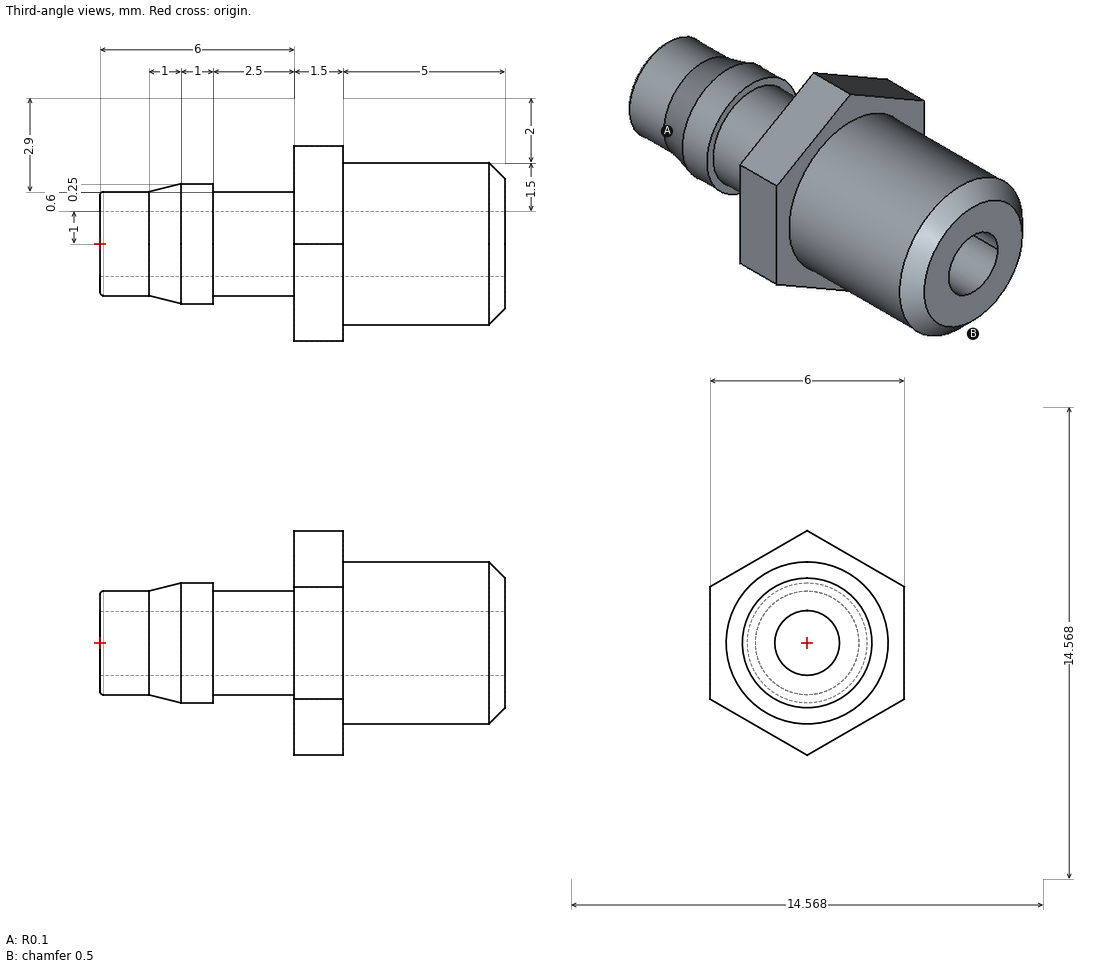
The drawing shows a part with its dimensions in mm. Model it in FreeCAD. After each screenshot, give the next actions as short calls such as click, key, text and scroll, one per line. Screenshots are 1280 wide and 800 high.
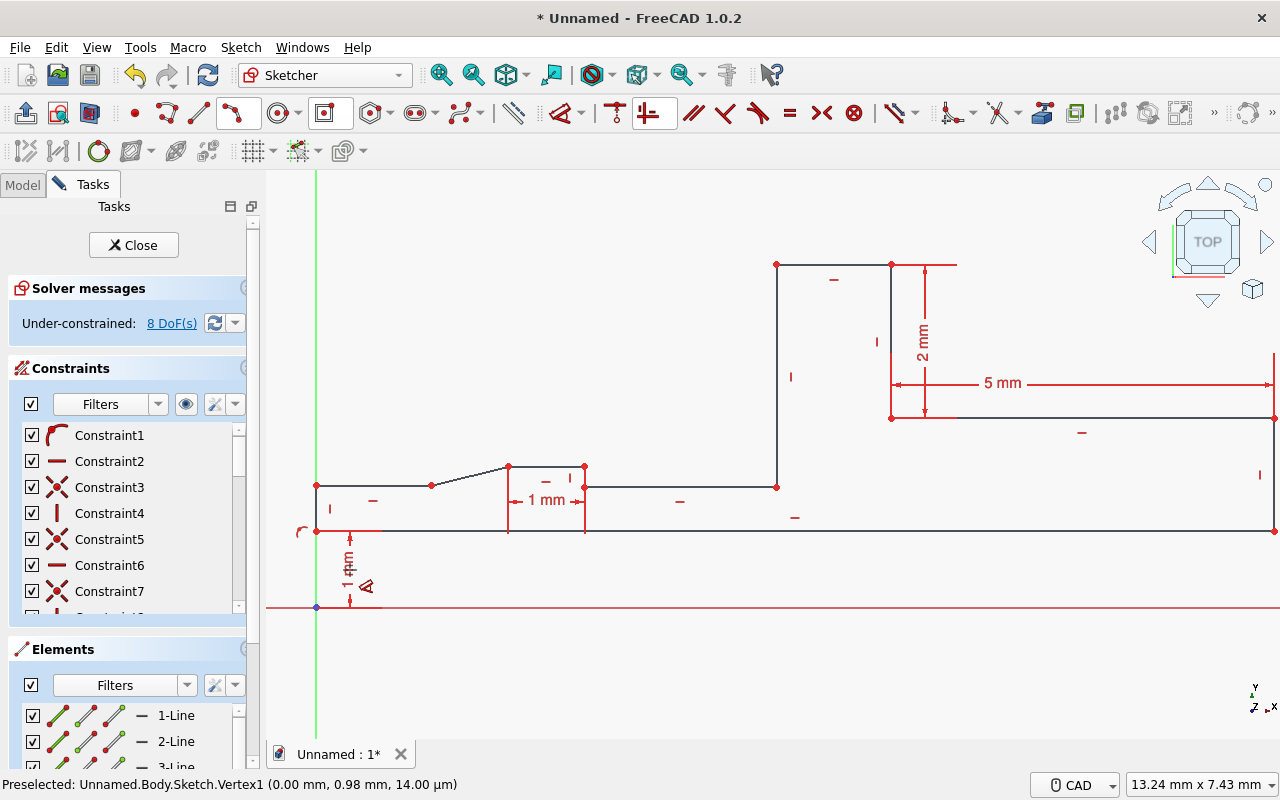
click(777, 265)
click(547, 642)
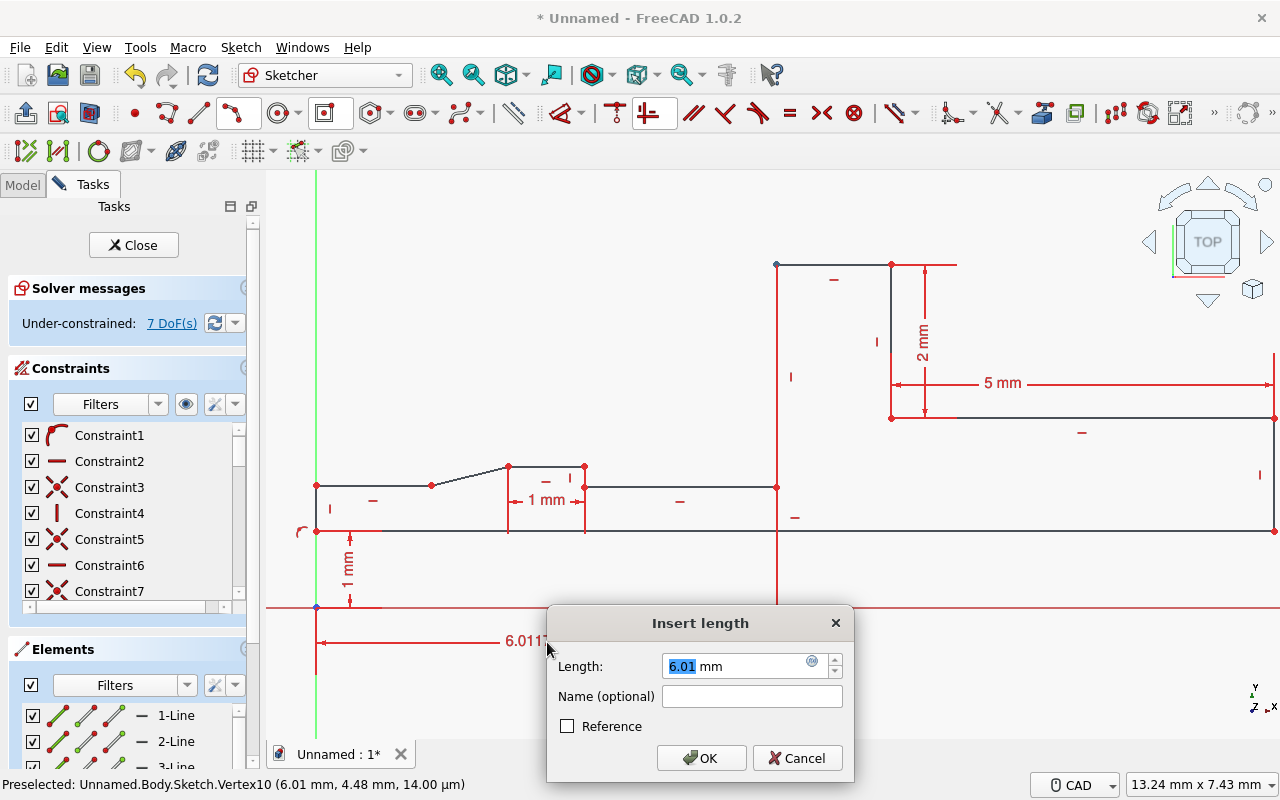
text(6)
key(Return)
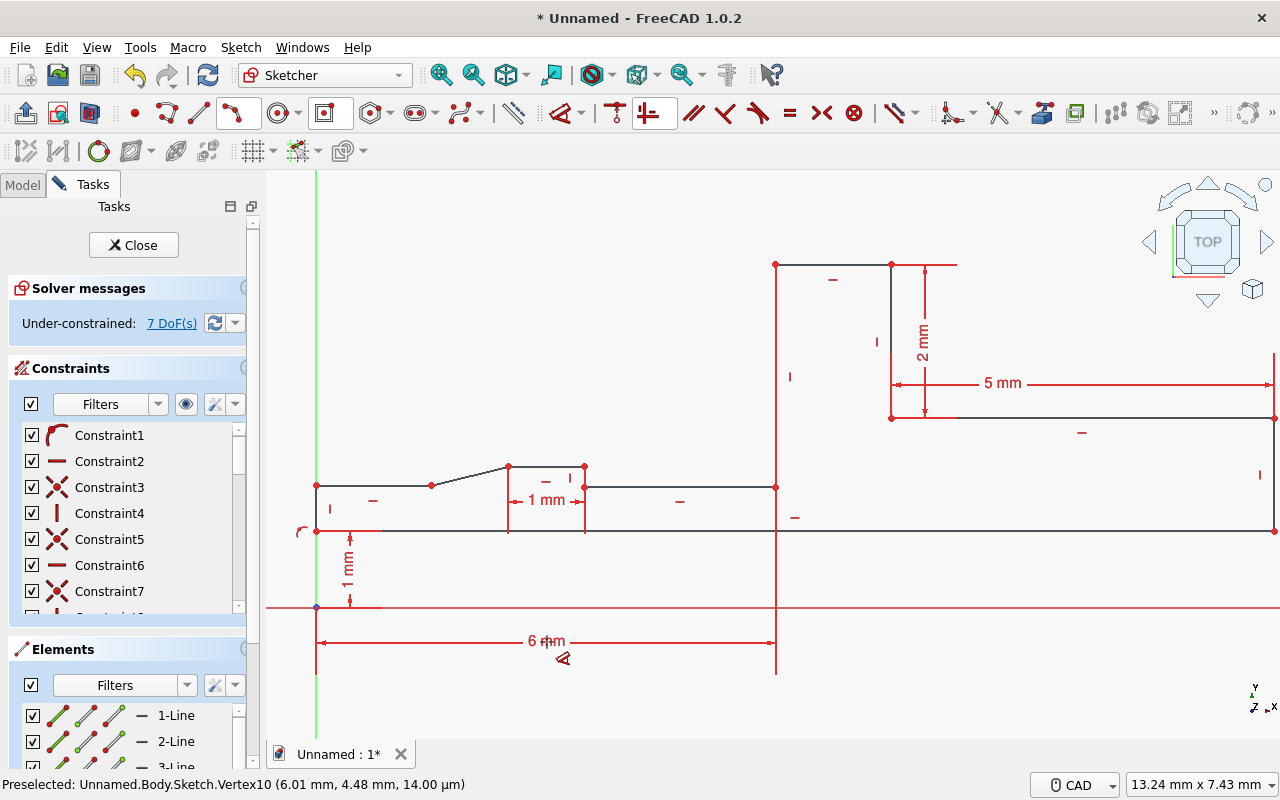
click(485, 473)
click(469, 433)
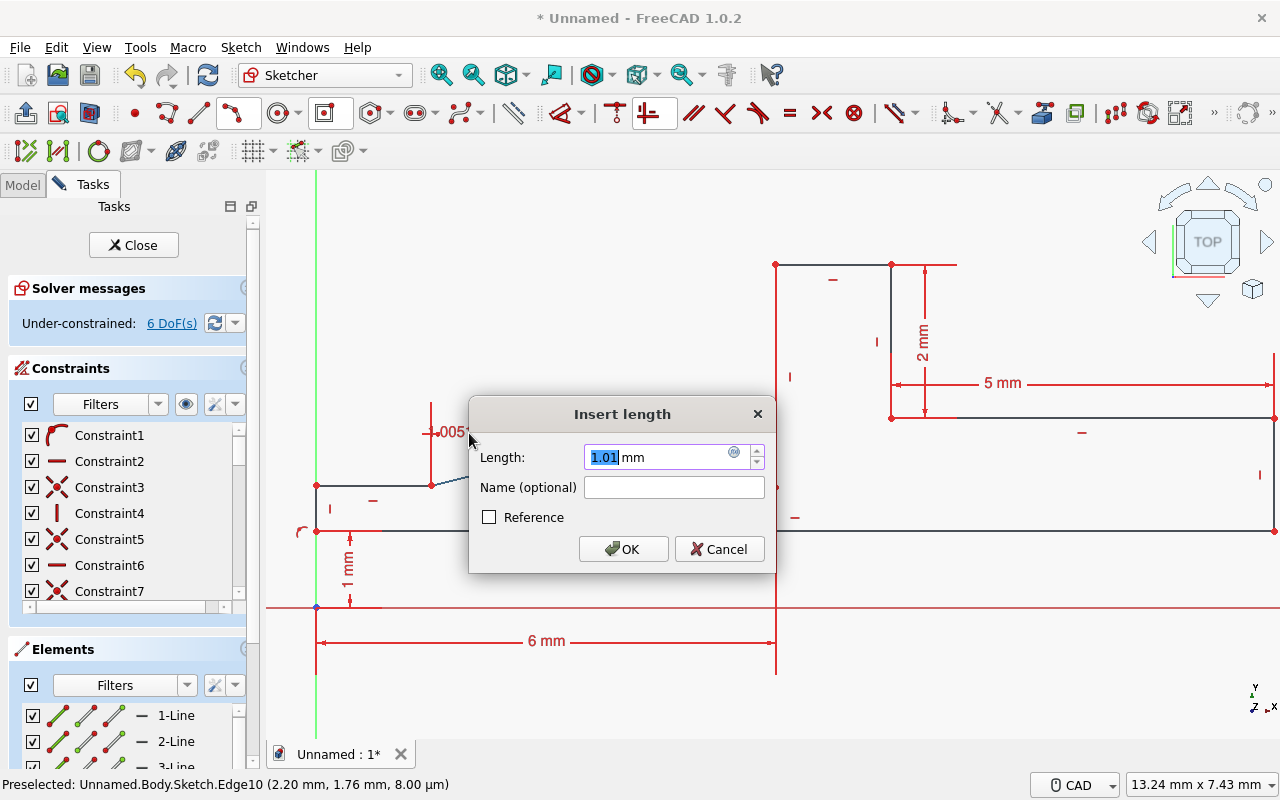
text(1)
key(Return)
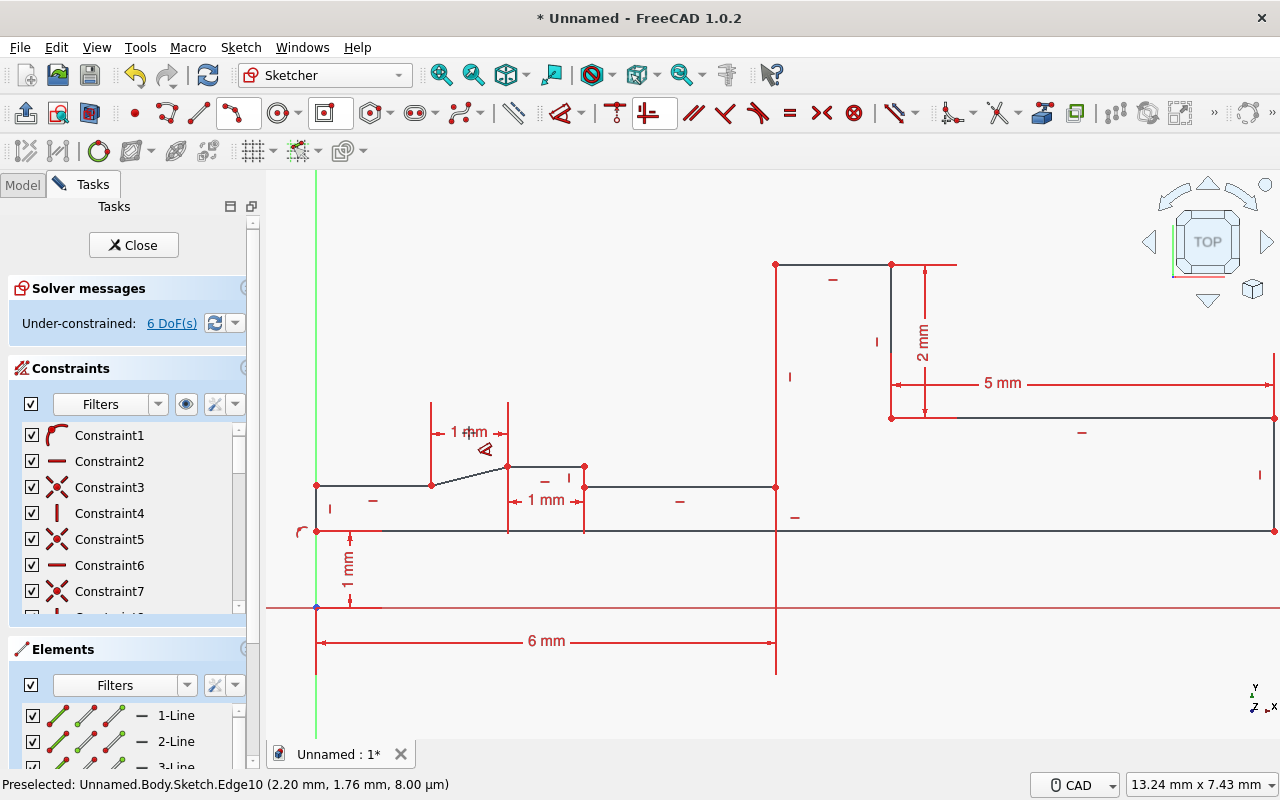
scroll(594, 478, down, 3)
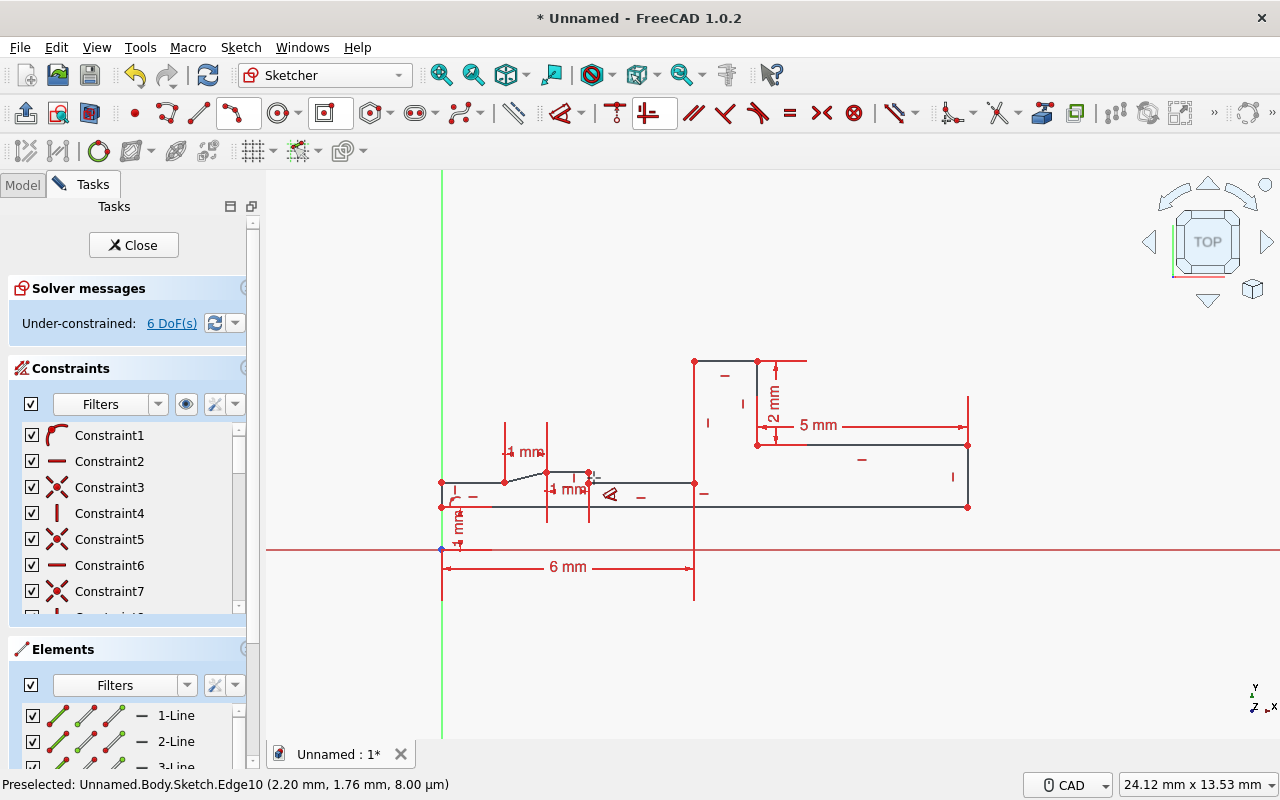
click(968, 489)
click(1002, 476)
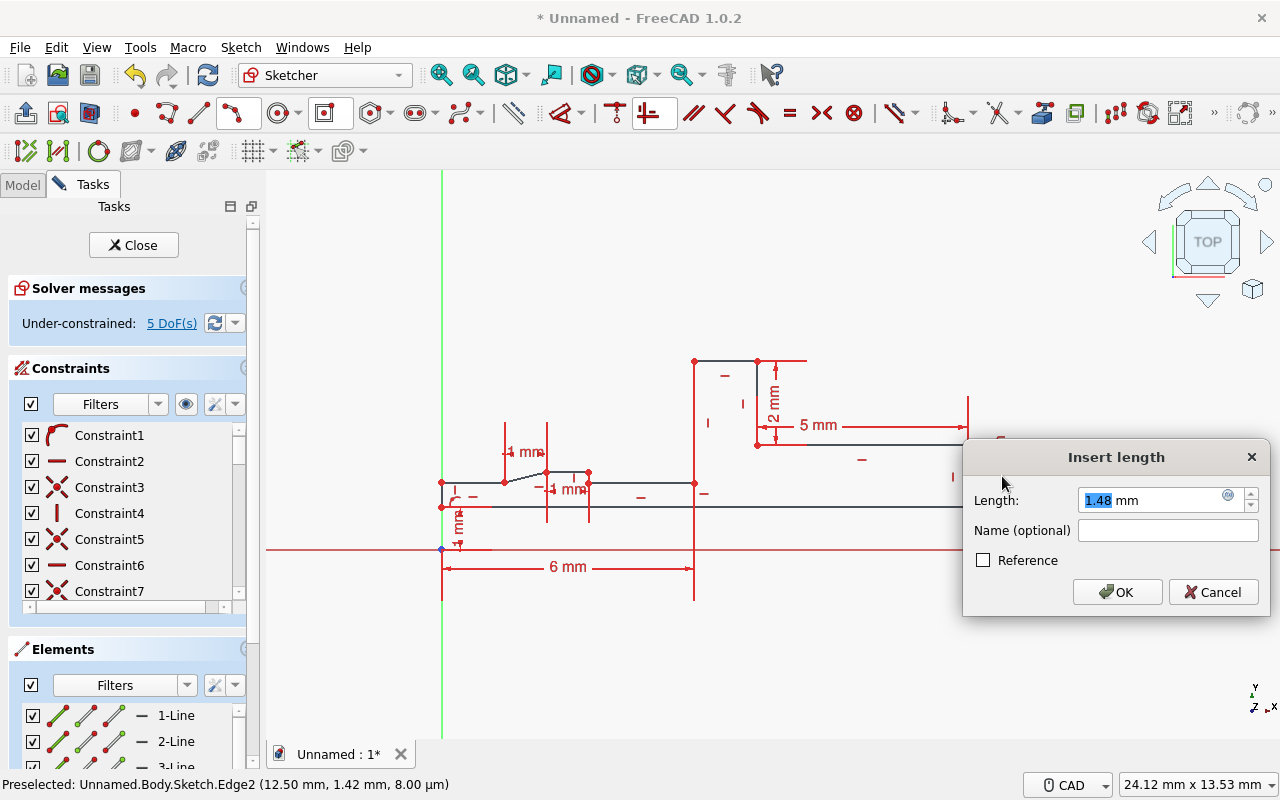
text(1.5)
key(Return)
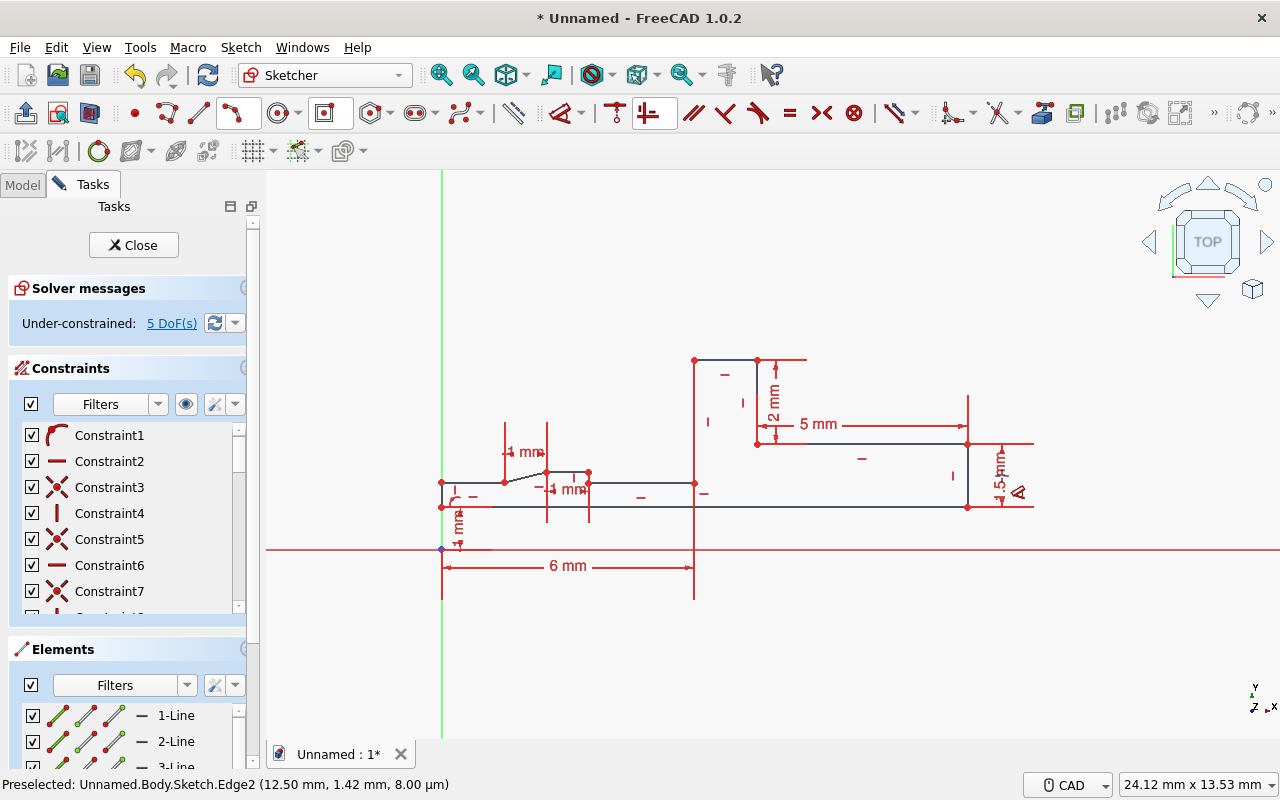
click(738, 360)
click(726, 326)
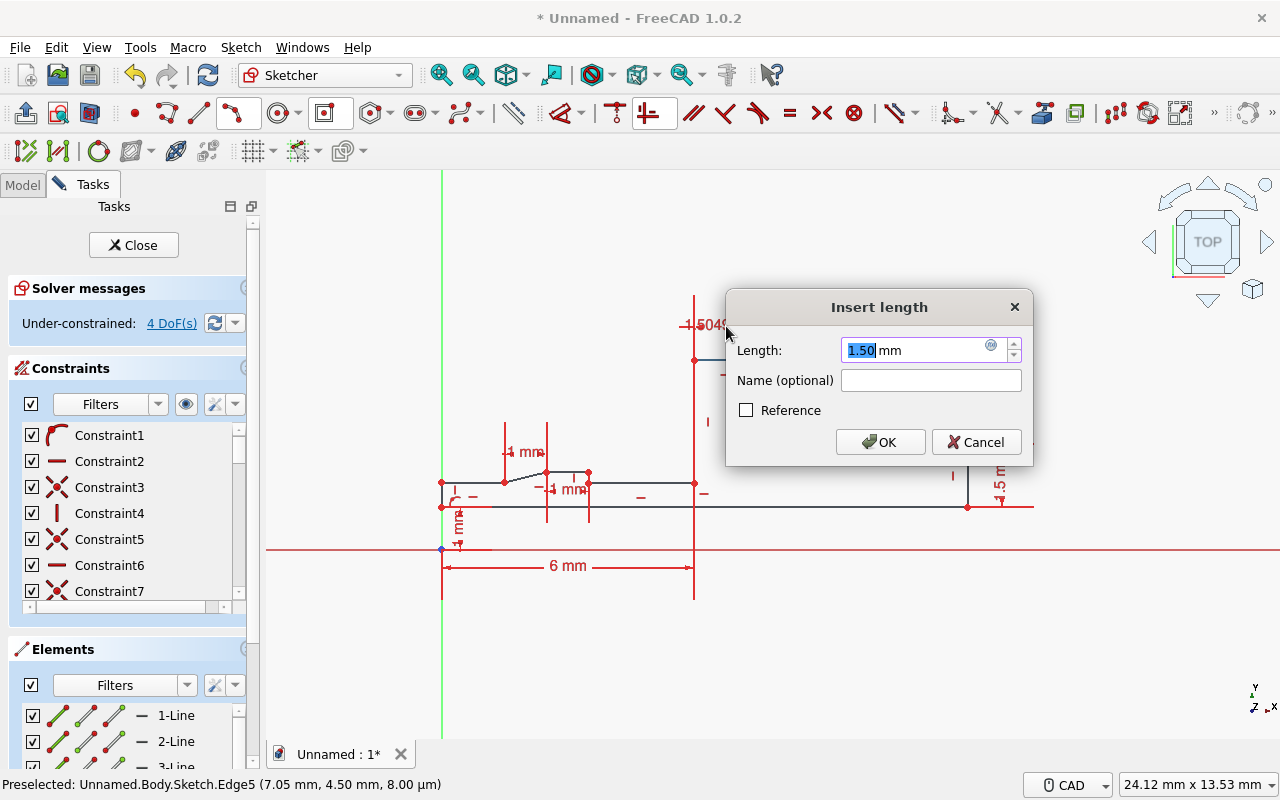
text(1.5)
key(Return)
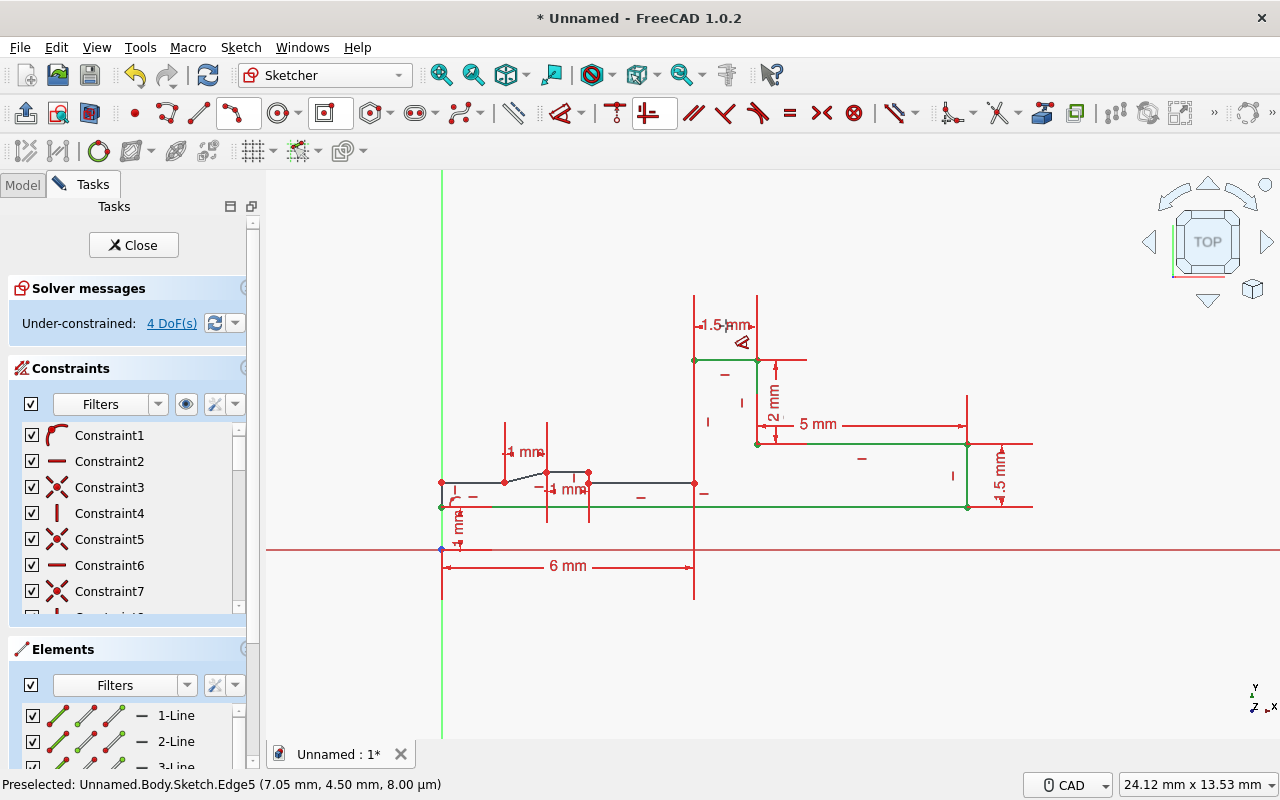
click(694, 397)
click(660, 422)